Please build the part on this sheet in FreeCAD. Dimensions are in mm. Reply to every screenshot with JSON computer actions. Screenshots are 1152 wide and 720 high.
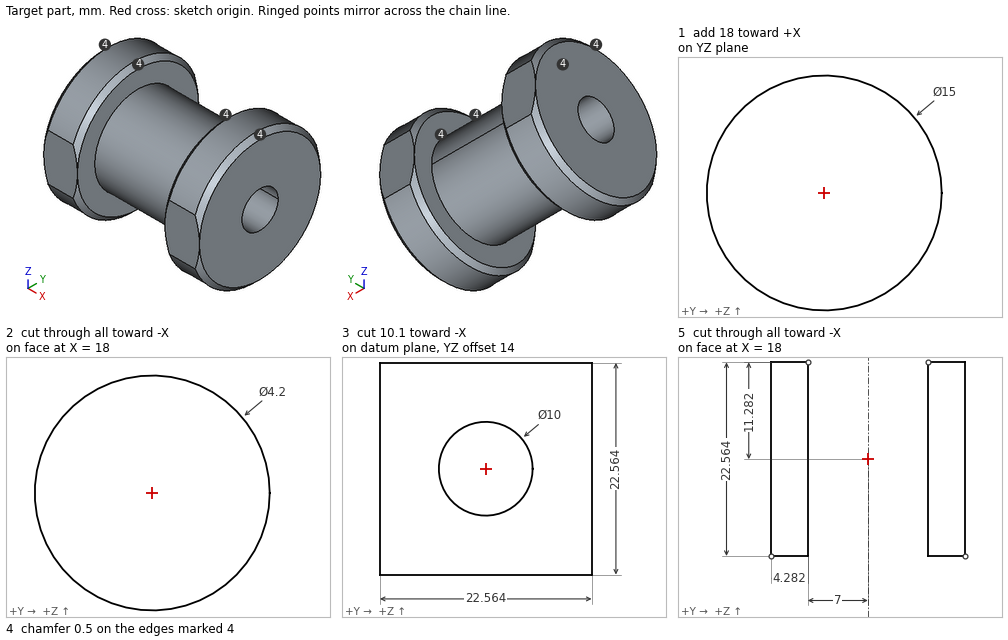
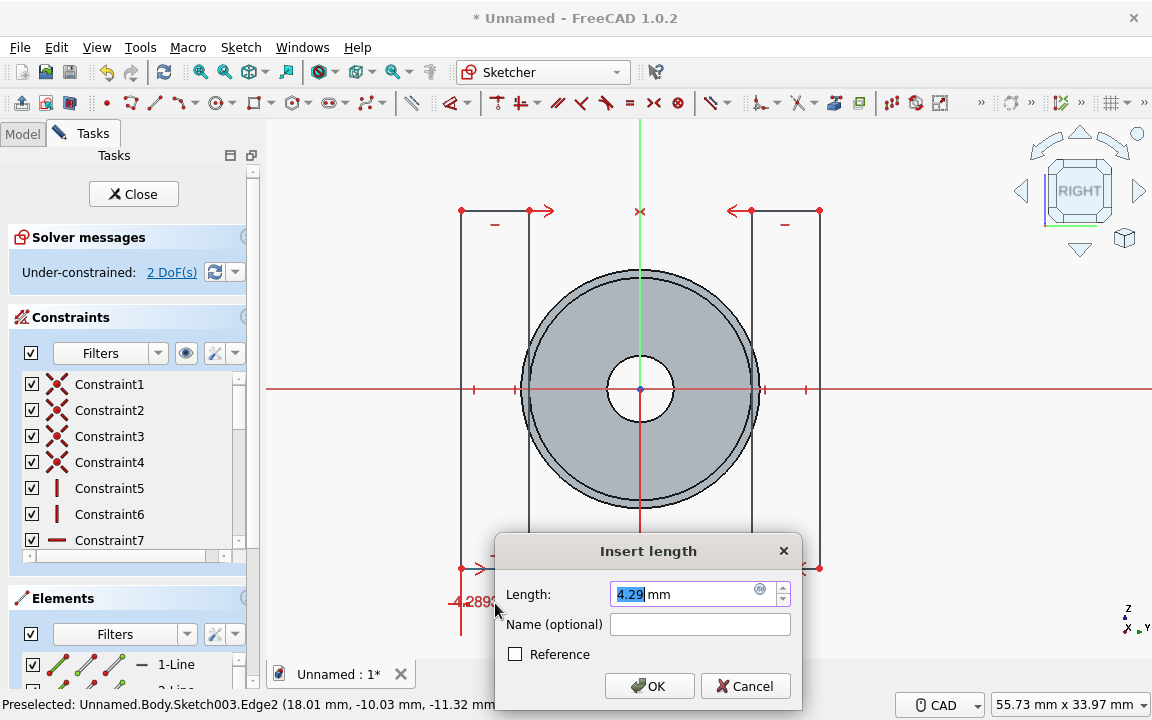
{"action": "type", "text": "4.282"}
{"action": "key", "text": "Return"}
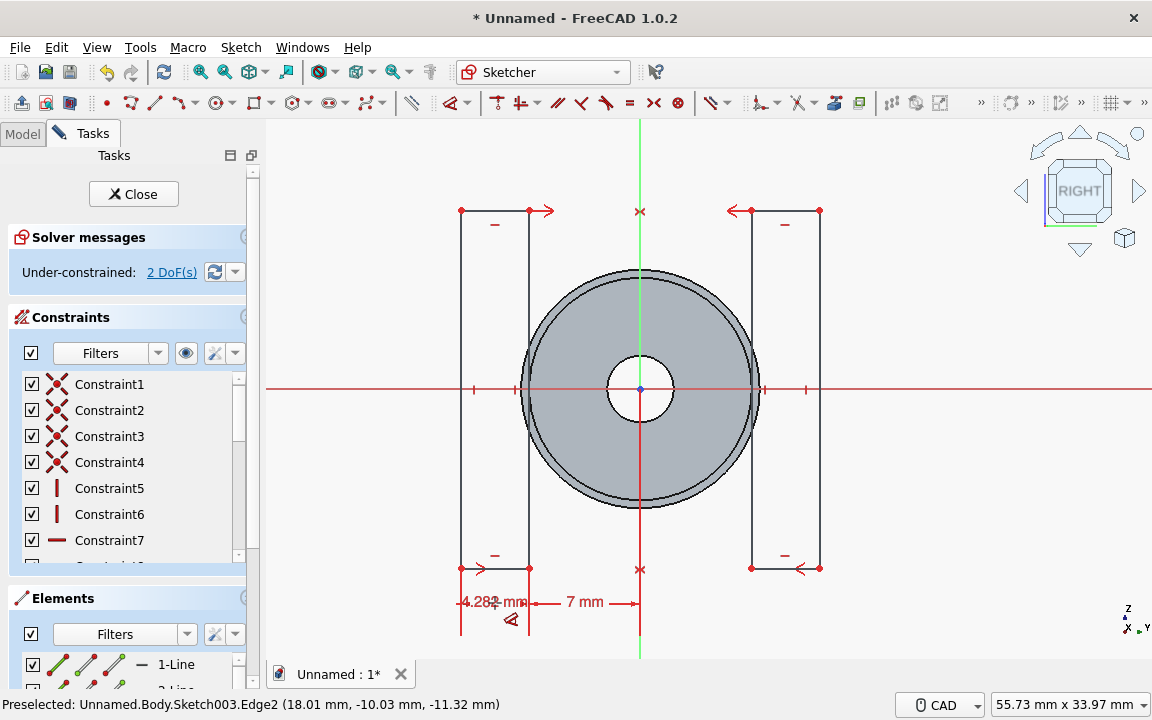
{"action": "left_click", "coordinate": [461, 318]}
{"action": "left_click", "coordinate": [427, 308]}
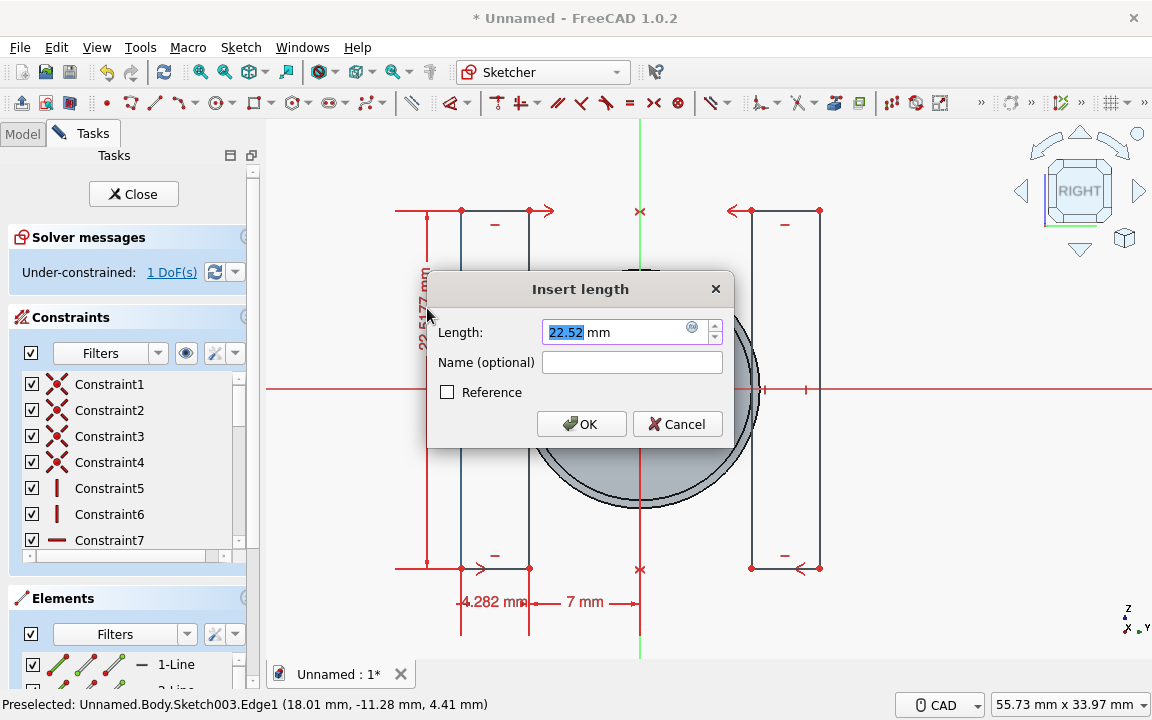
{"action": "type", "text": "22.564"}
{"action": "key", "text": "Return"}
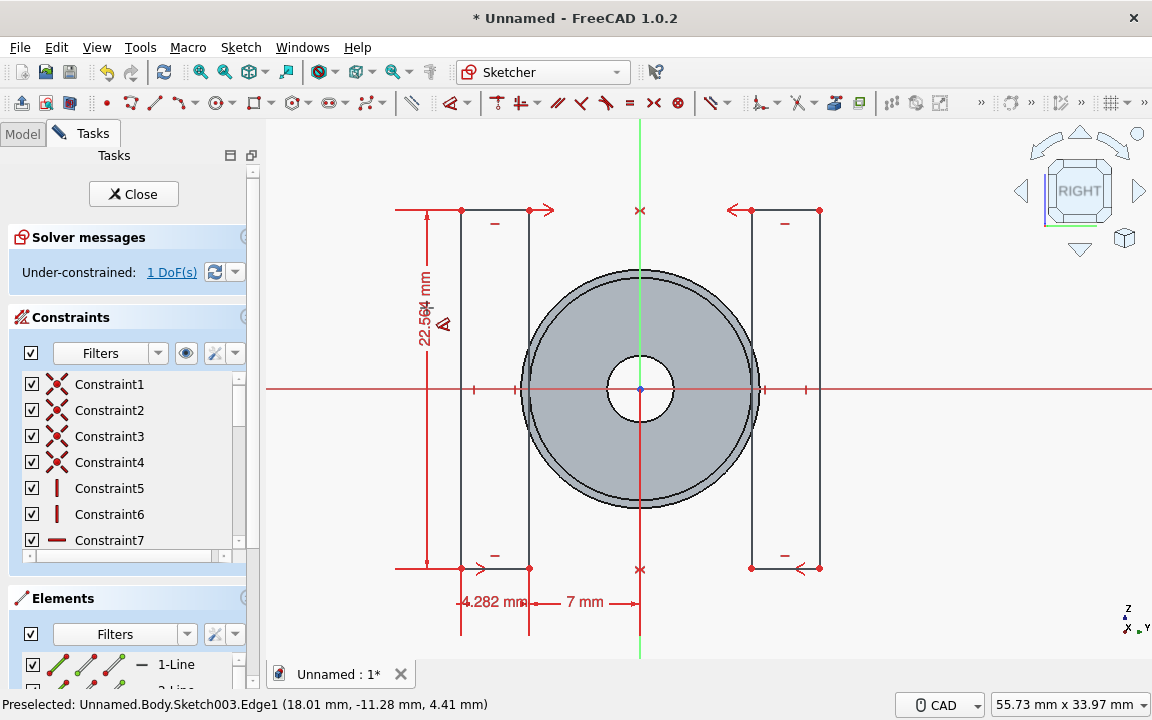
{"action": "left_click", "coordinate": [461, 210]}
{"action": "left_click", "coordinate": [427, 259]}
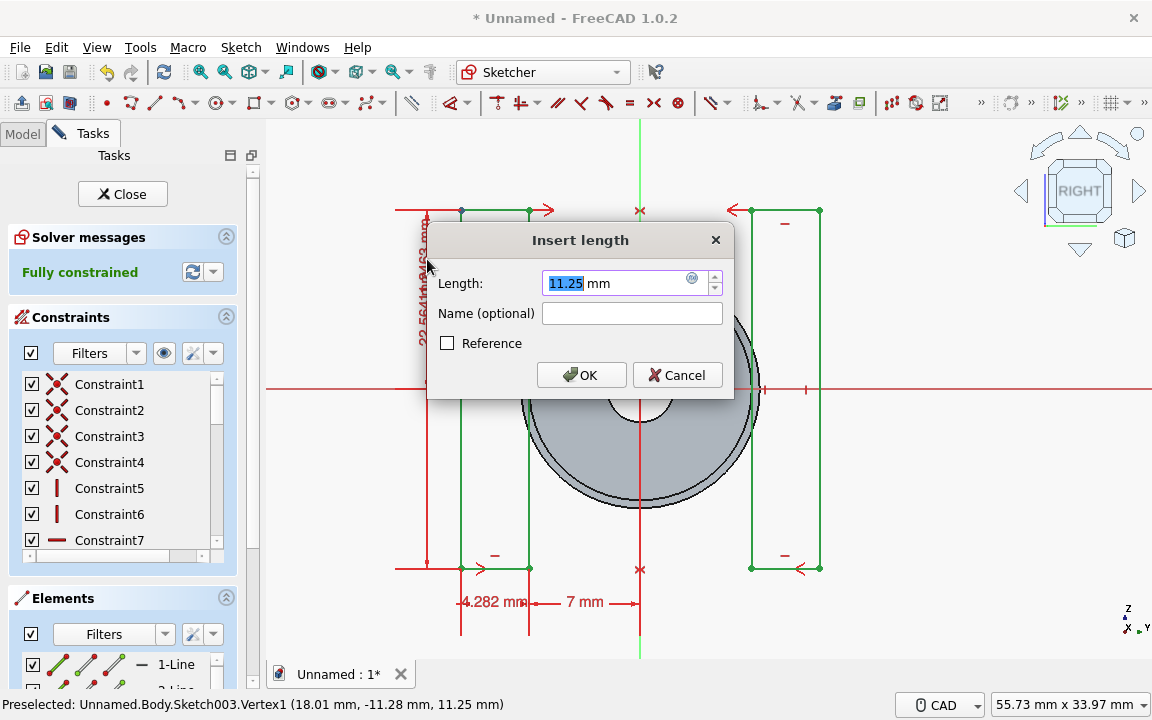
{"action": "type", "text": "11.282"}
{"action": "key", "text": "Return"}
{"action": "key", "text": "Escape"}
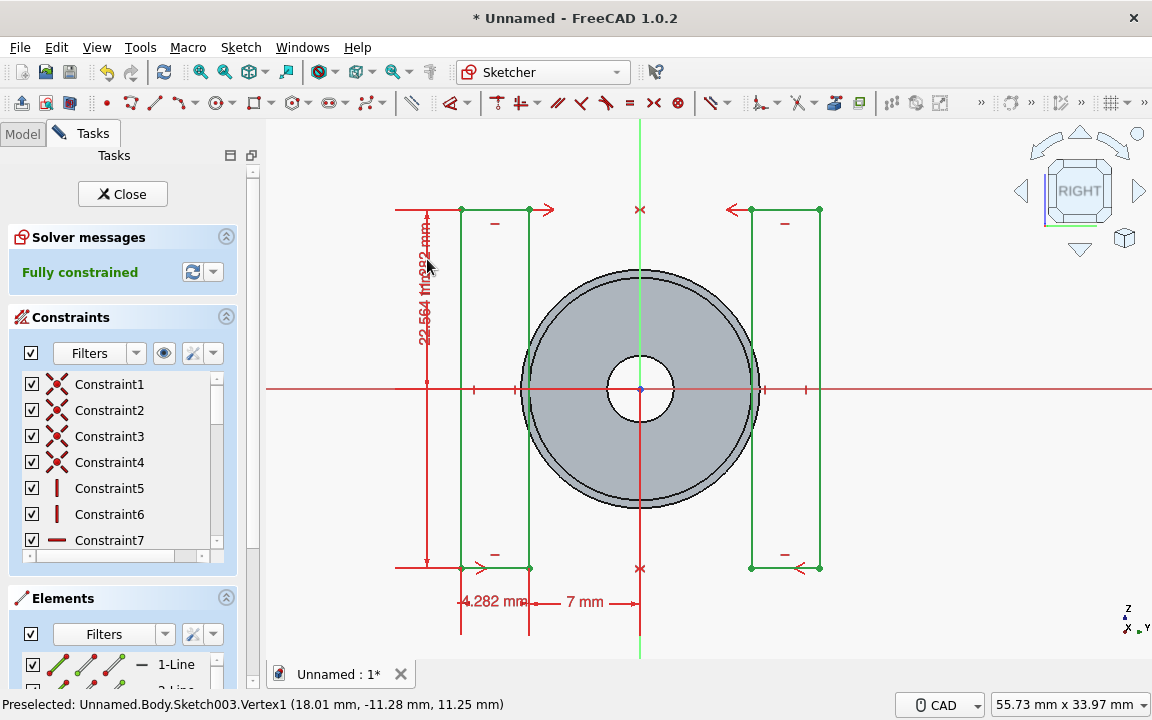
{"action": "left_click", "coordinate": [123, 194]}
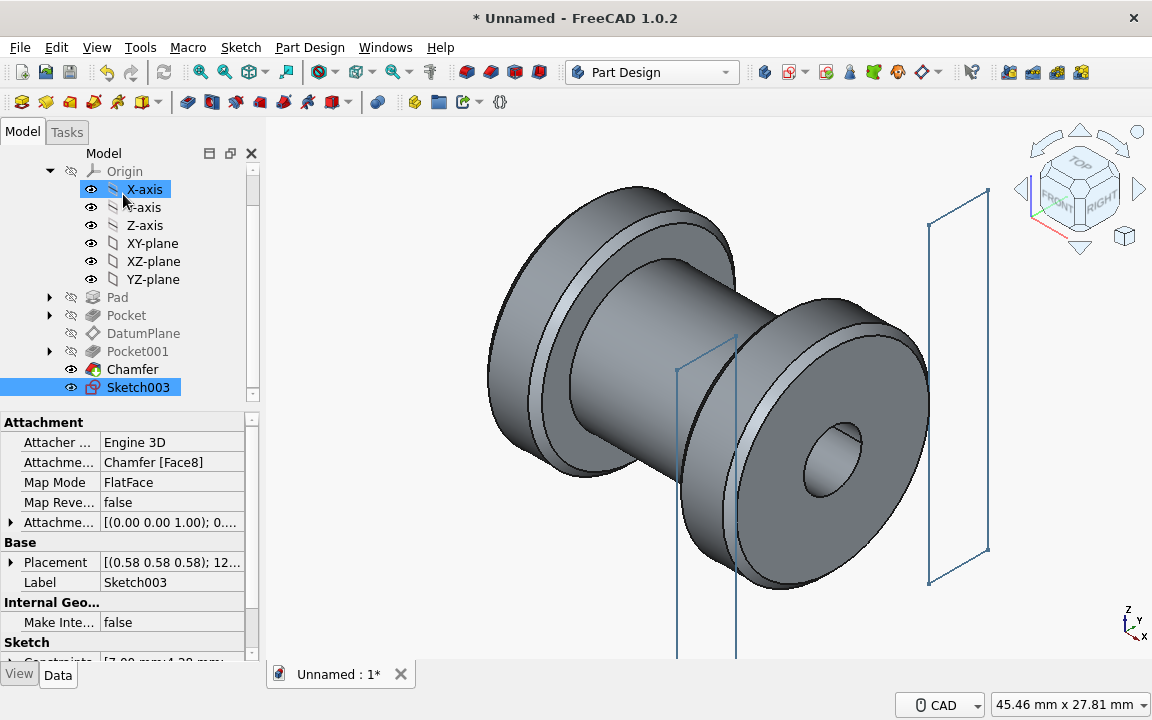
{"action": "left_click", "coordinate": [188, 102]}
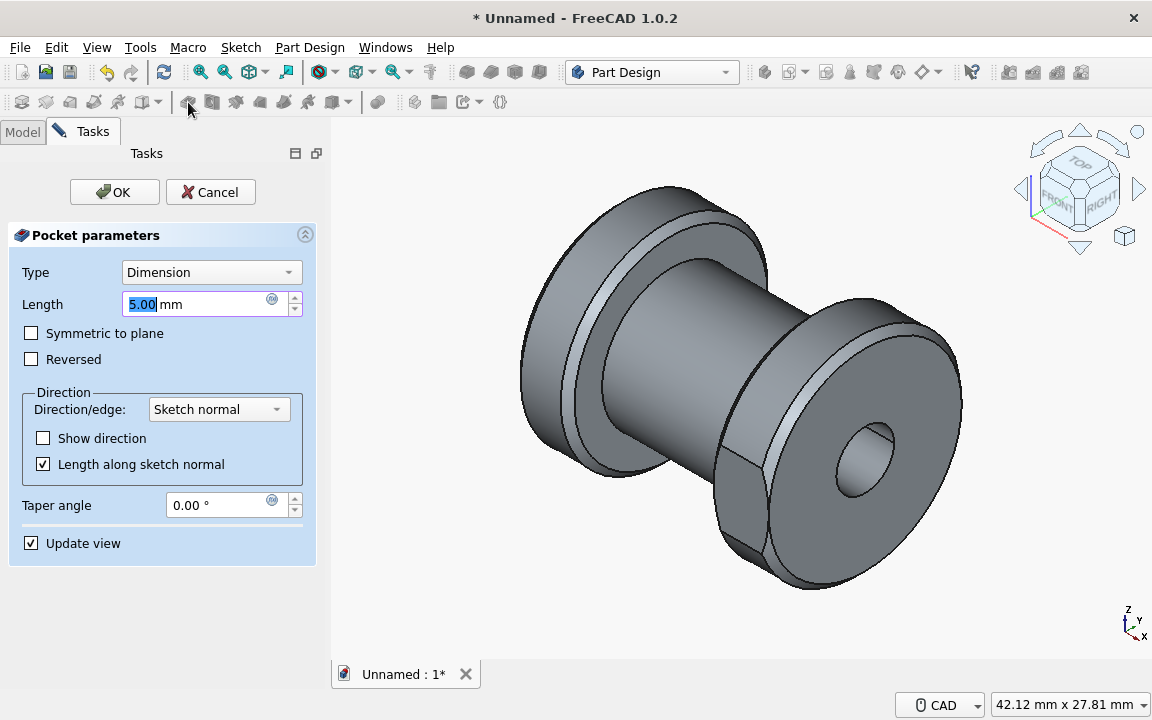
{"action": "left_click", "coordinate": [212, 272]}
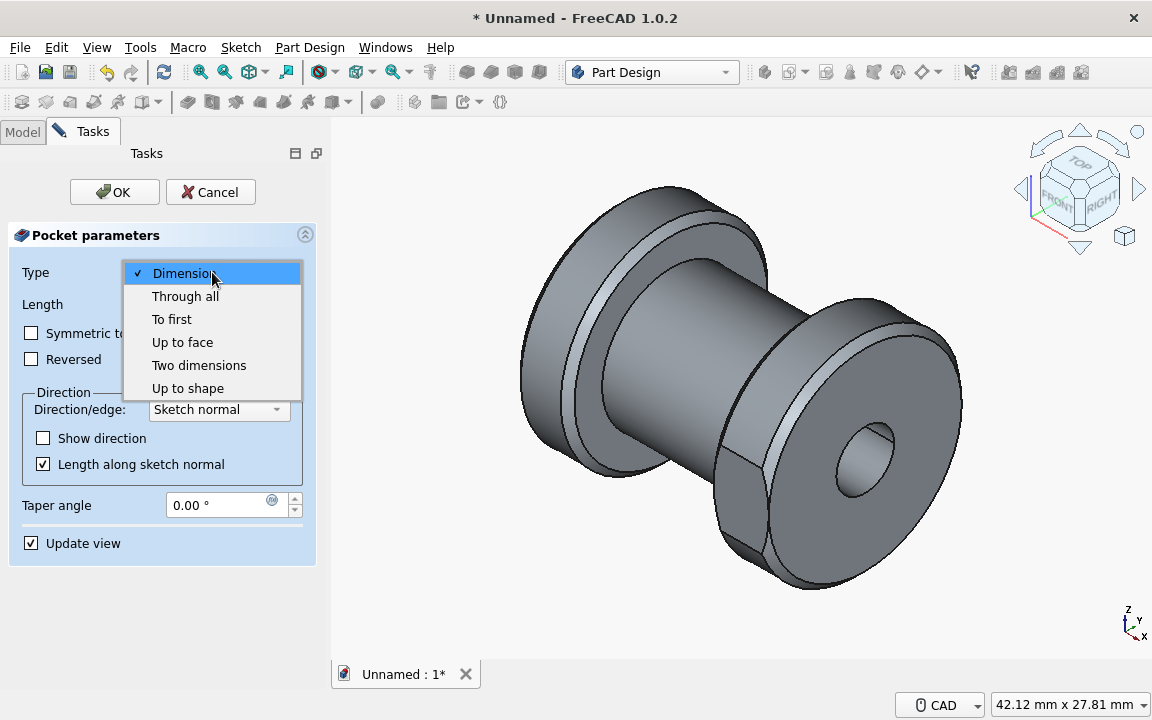
{"action": "left_click", "coordinate": [212, 296]}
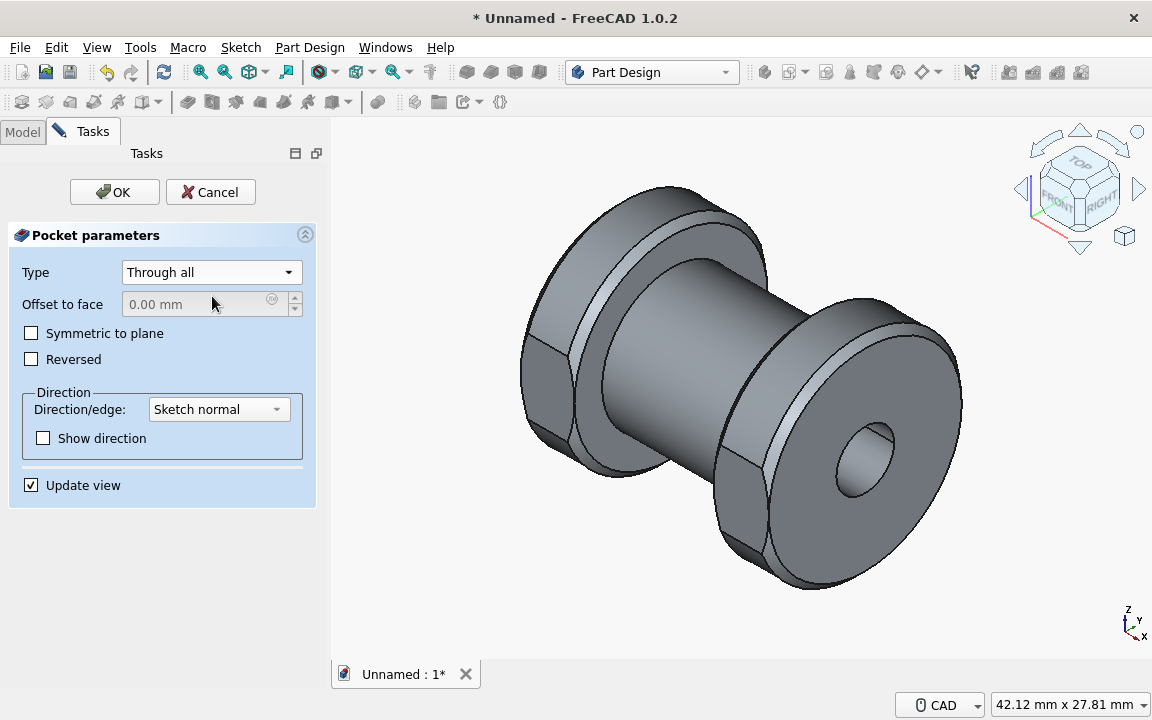
{"action": "left_click", "coordinate": [115, 192]}